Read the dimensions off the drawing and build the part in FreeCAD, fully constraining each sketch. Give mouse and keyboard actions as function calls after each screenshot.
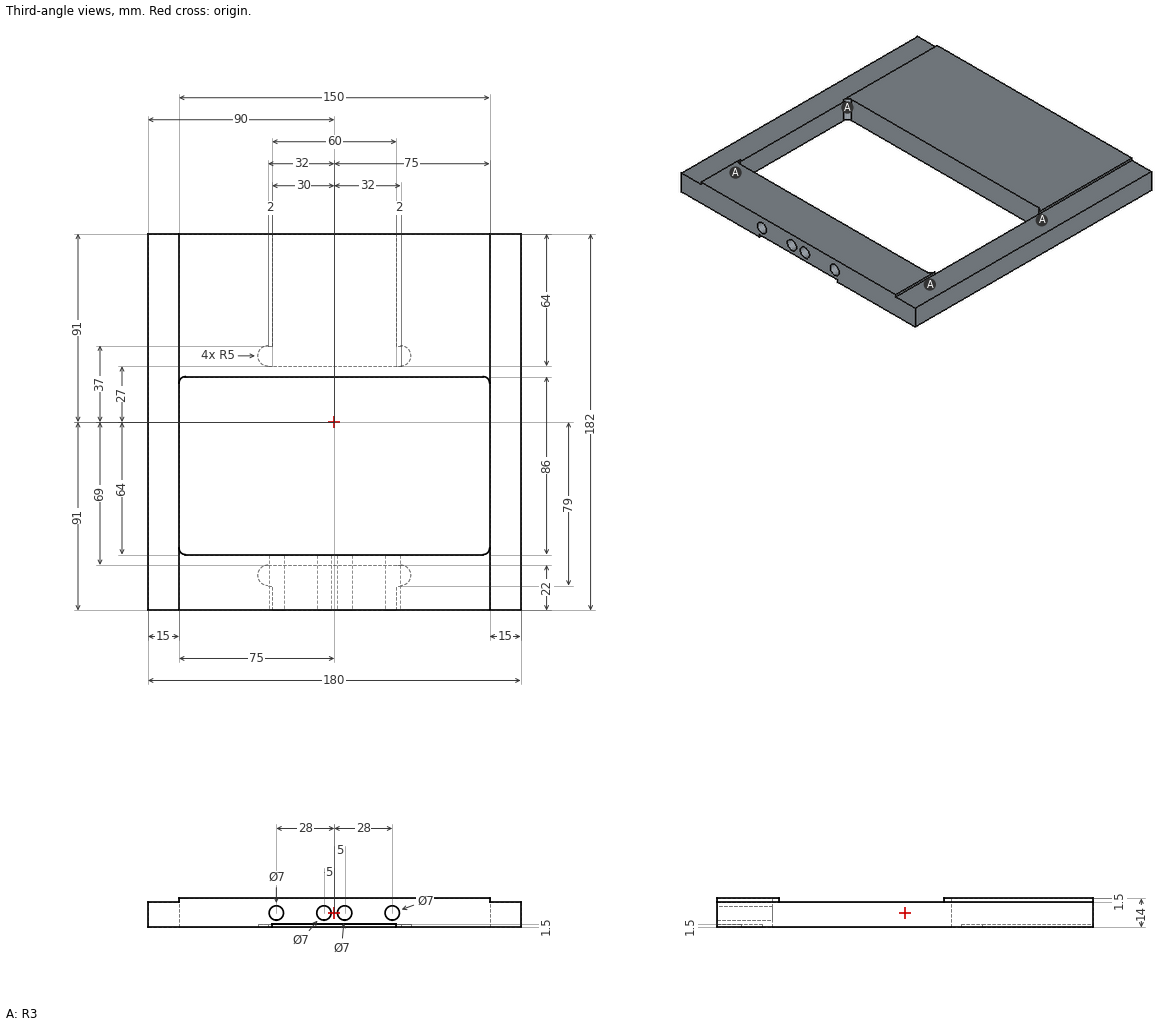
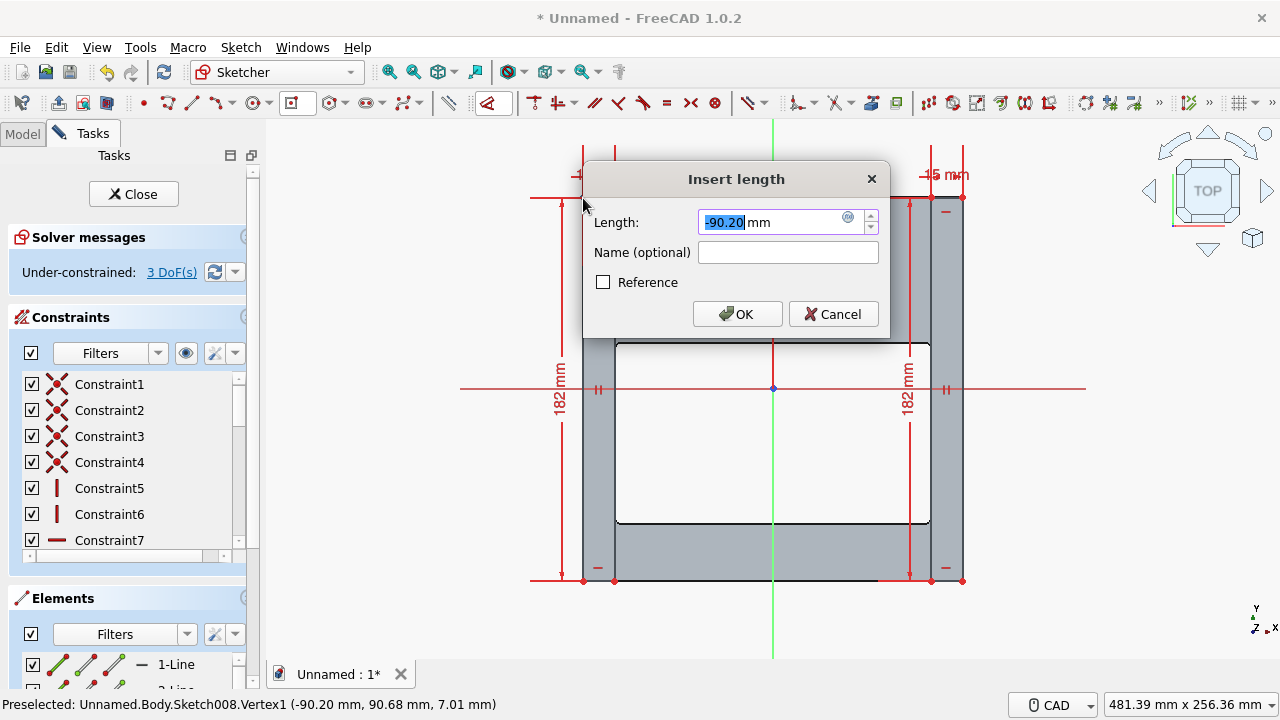
text(-90)
key(Return)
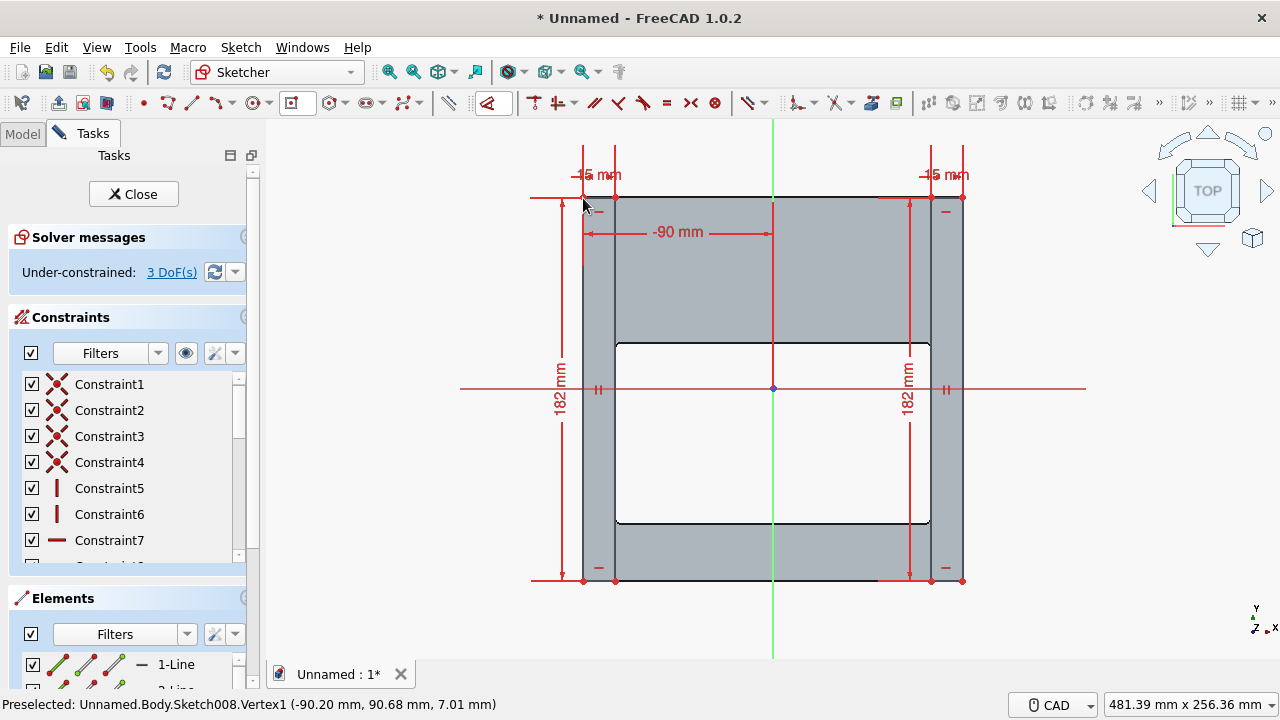
click(583, 198)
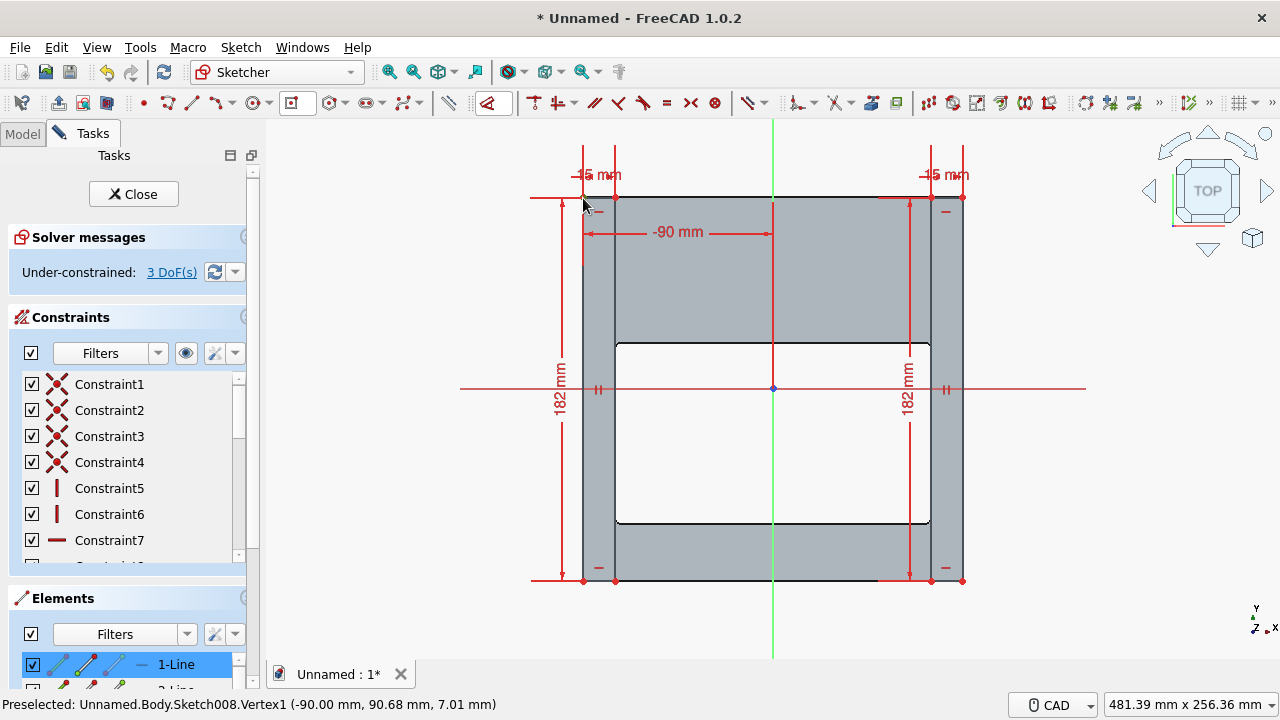
key(i)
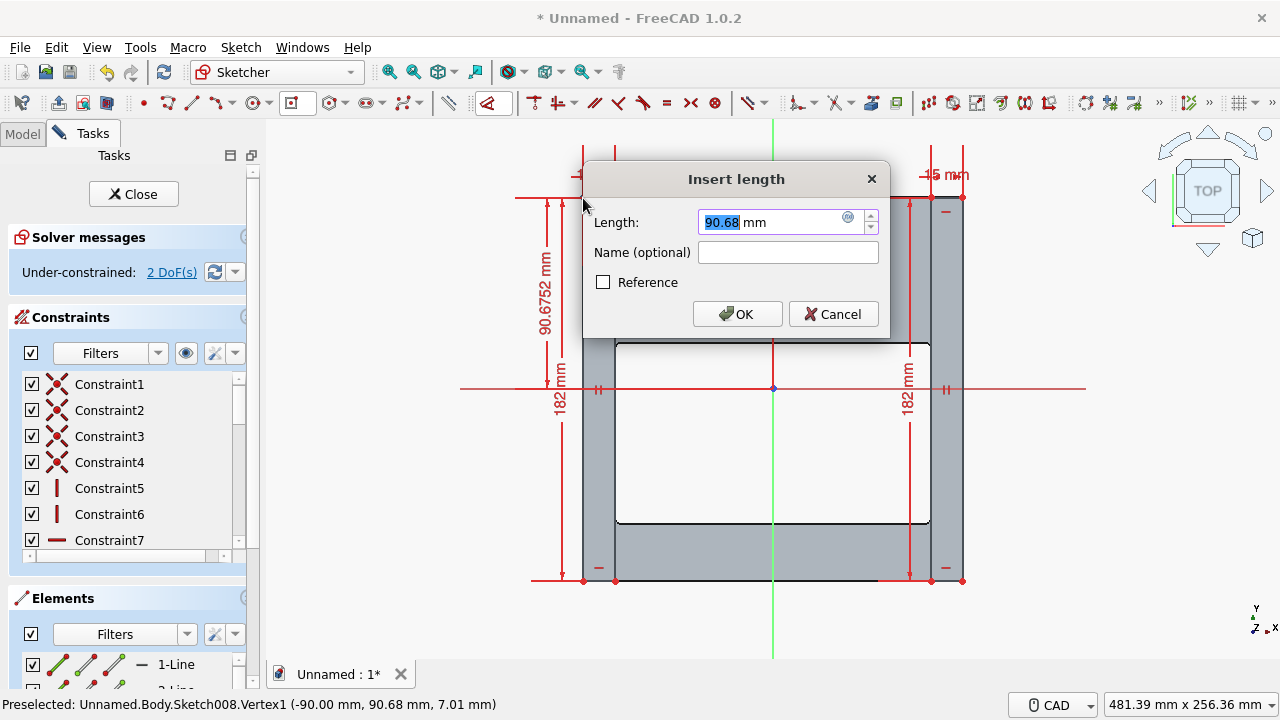
text(91)
key(Return)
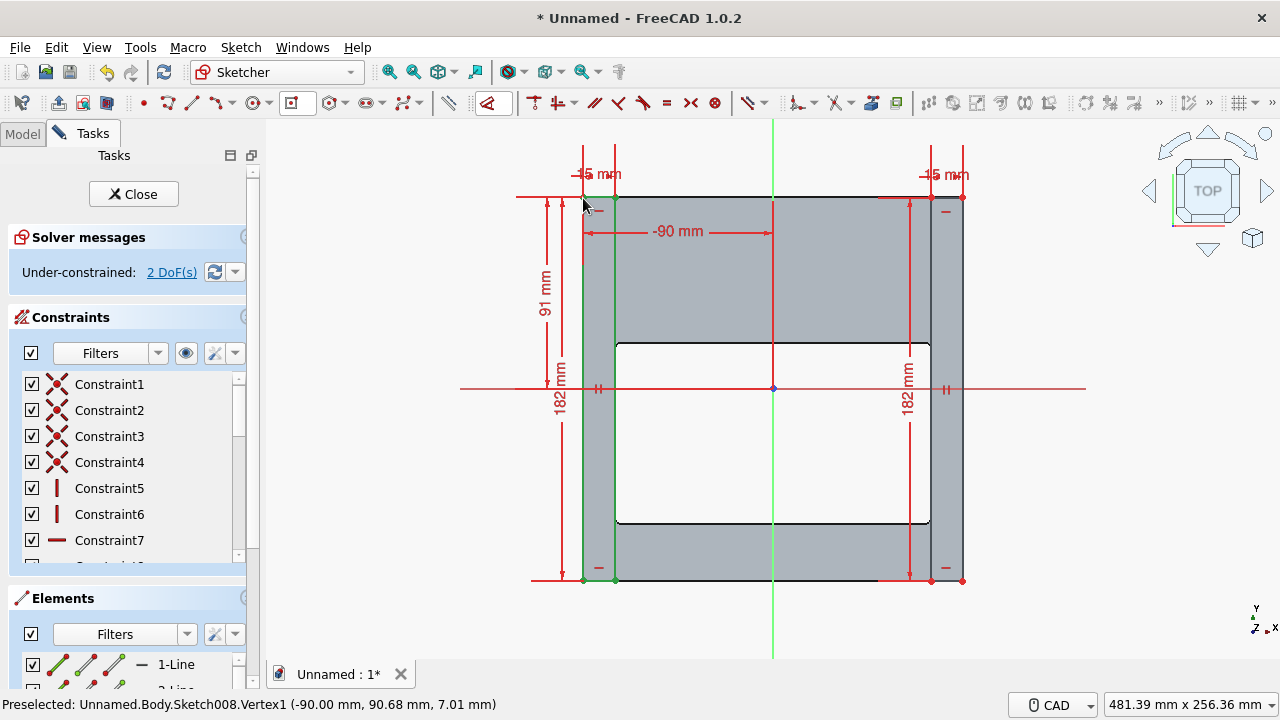
click(931, 198)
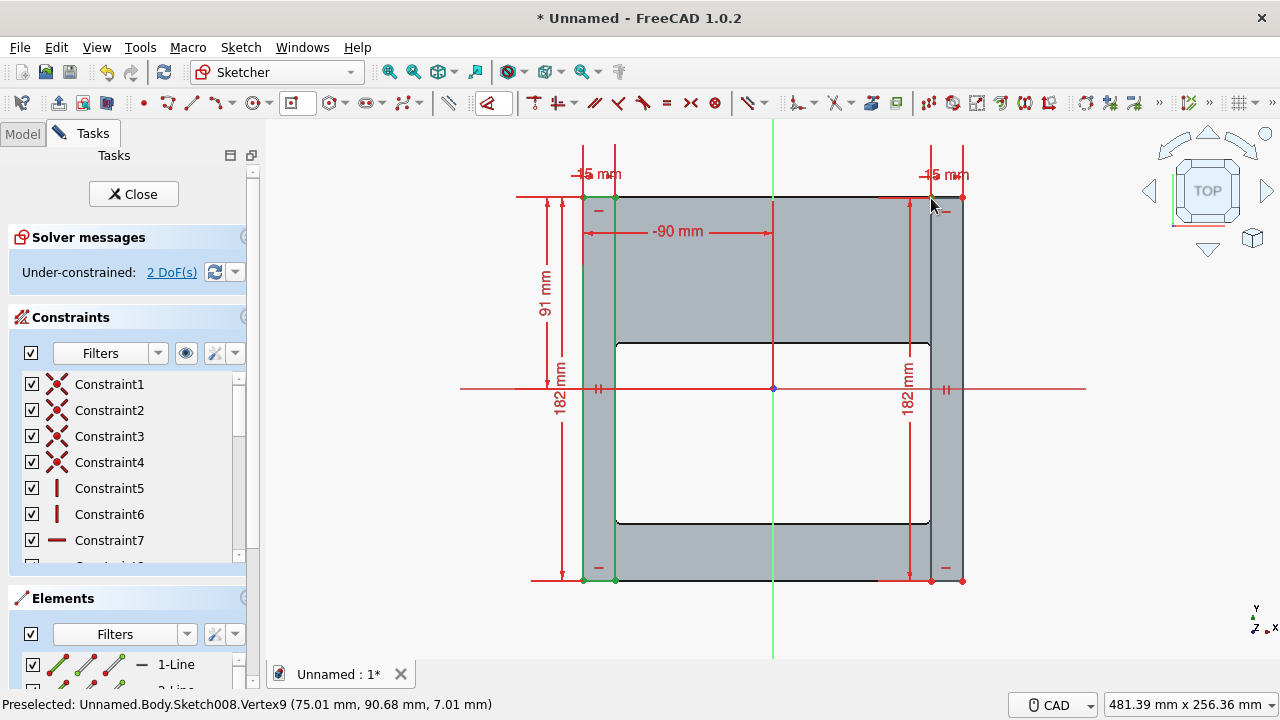
click(506, 104)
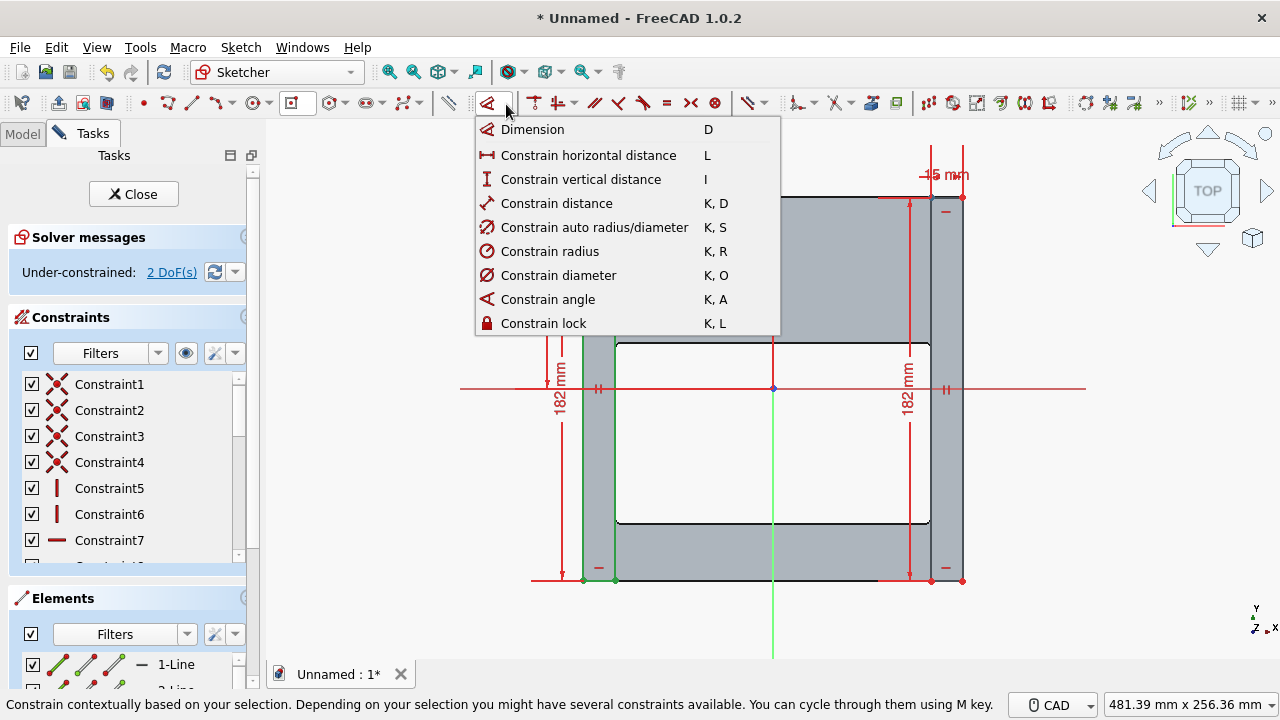
click(628, 155)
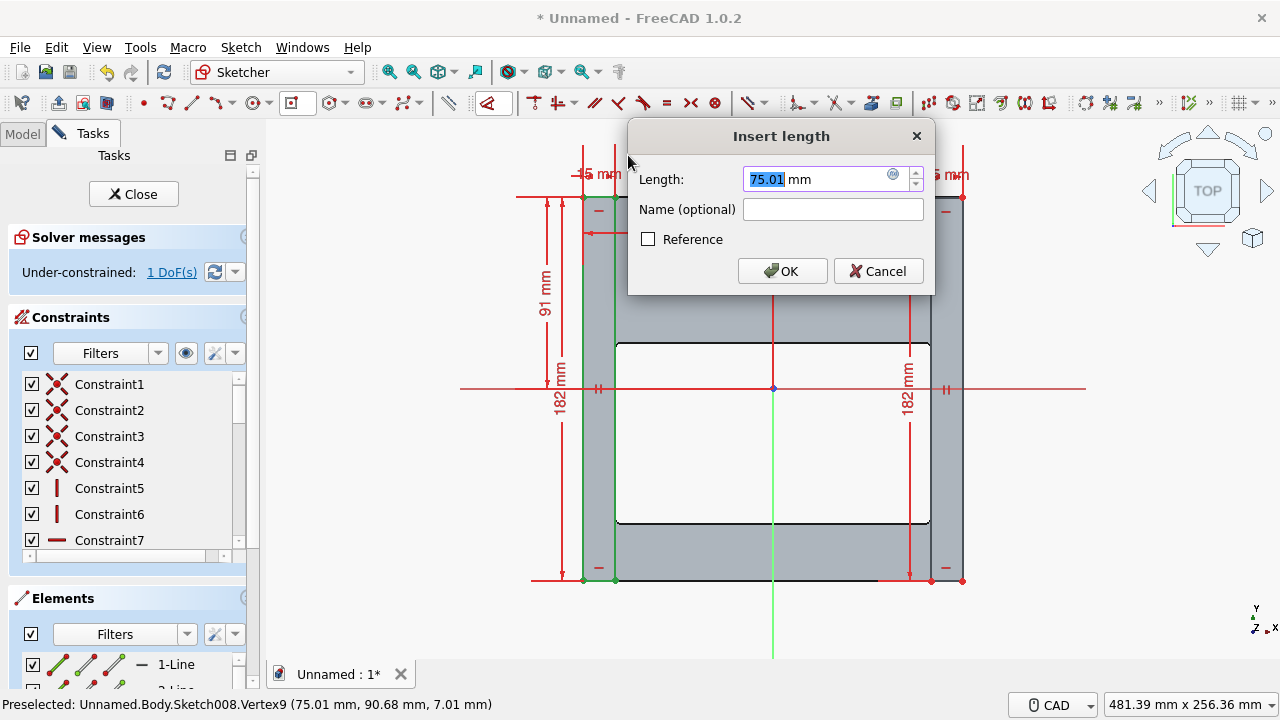
text(75)
key(Return)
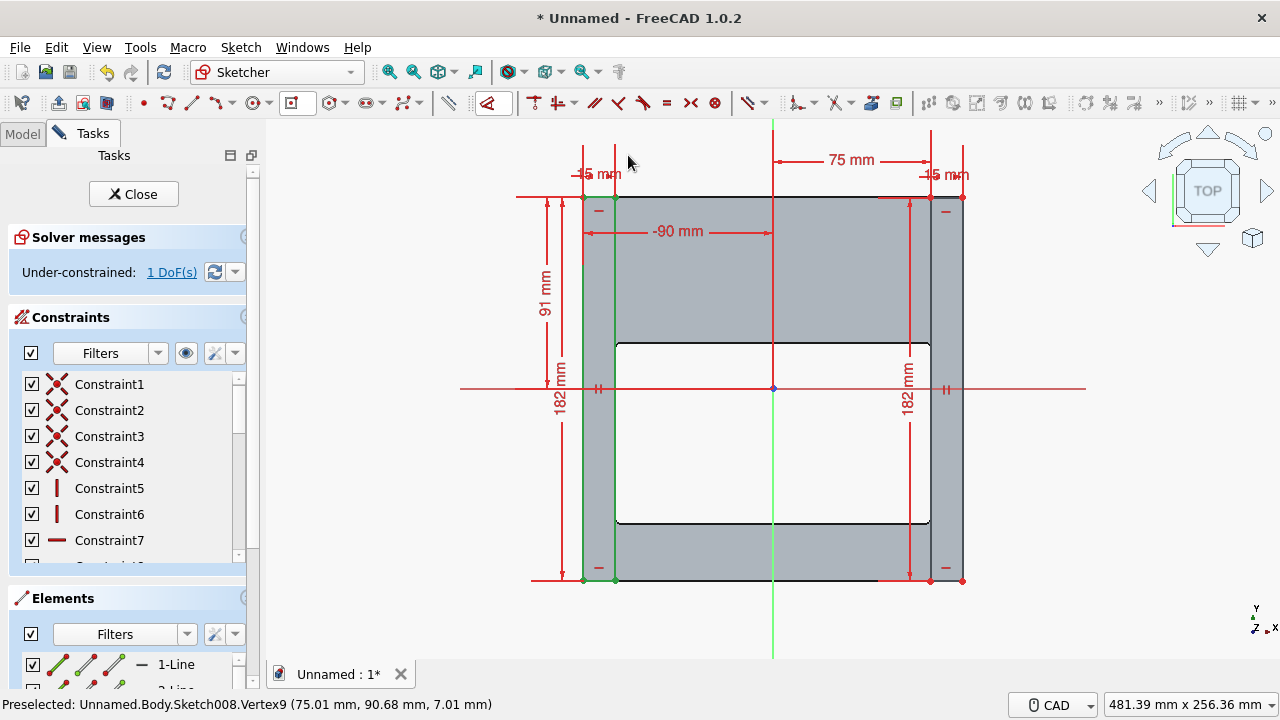
click(931, 198)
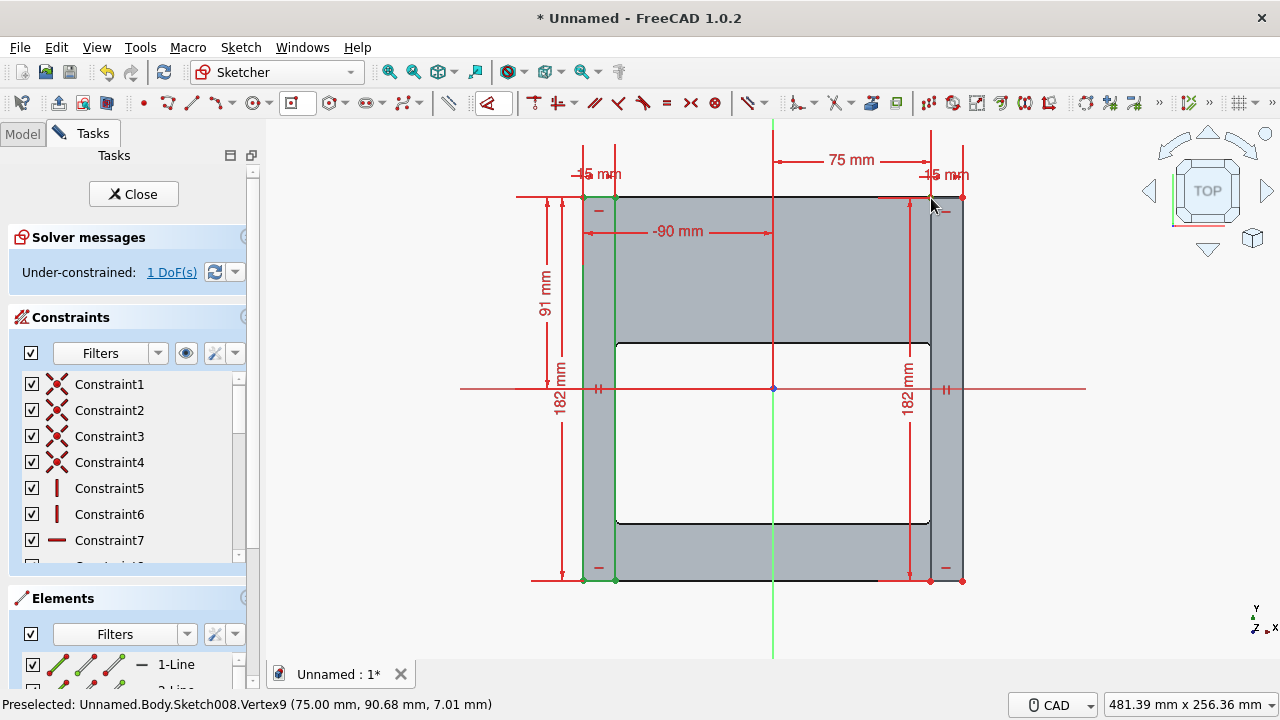
key(i)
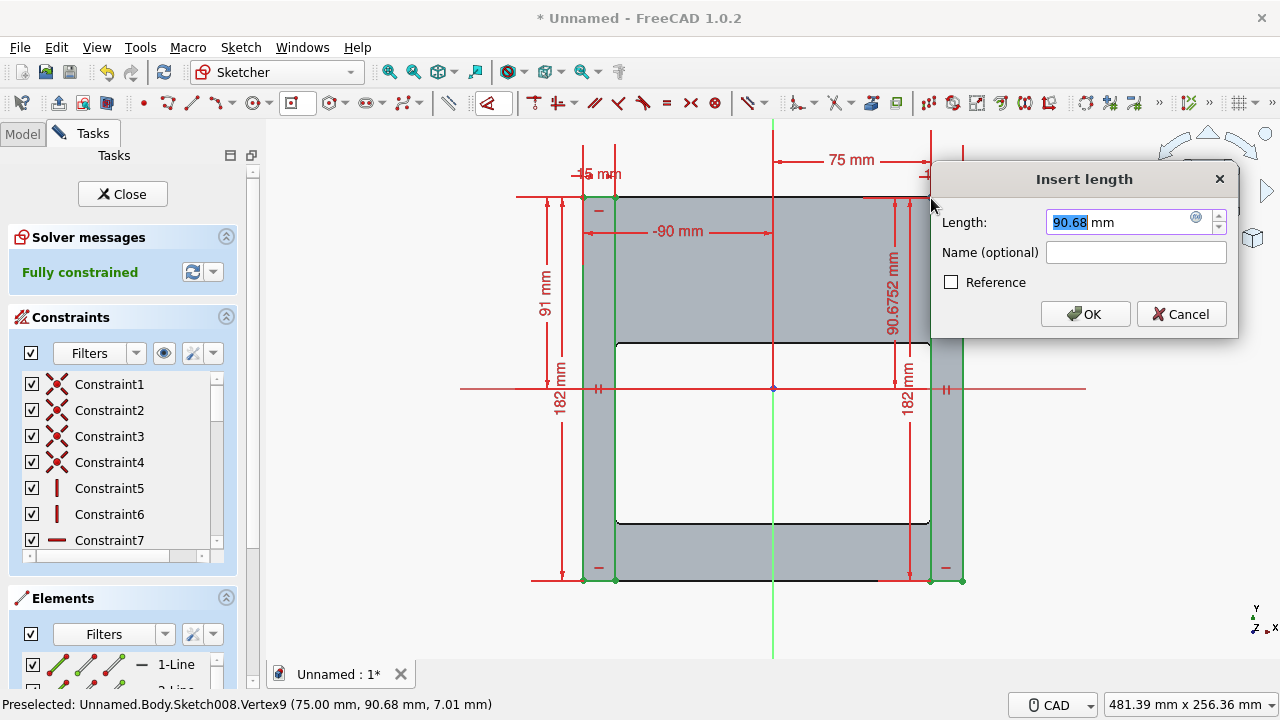
text(91)
key(Return)